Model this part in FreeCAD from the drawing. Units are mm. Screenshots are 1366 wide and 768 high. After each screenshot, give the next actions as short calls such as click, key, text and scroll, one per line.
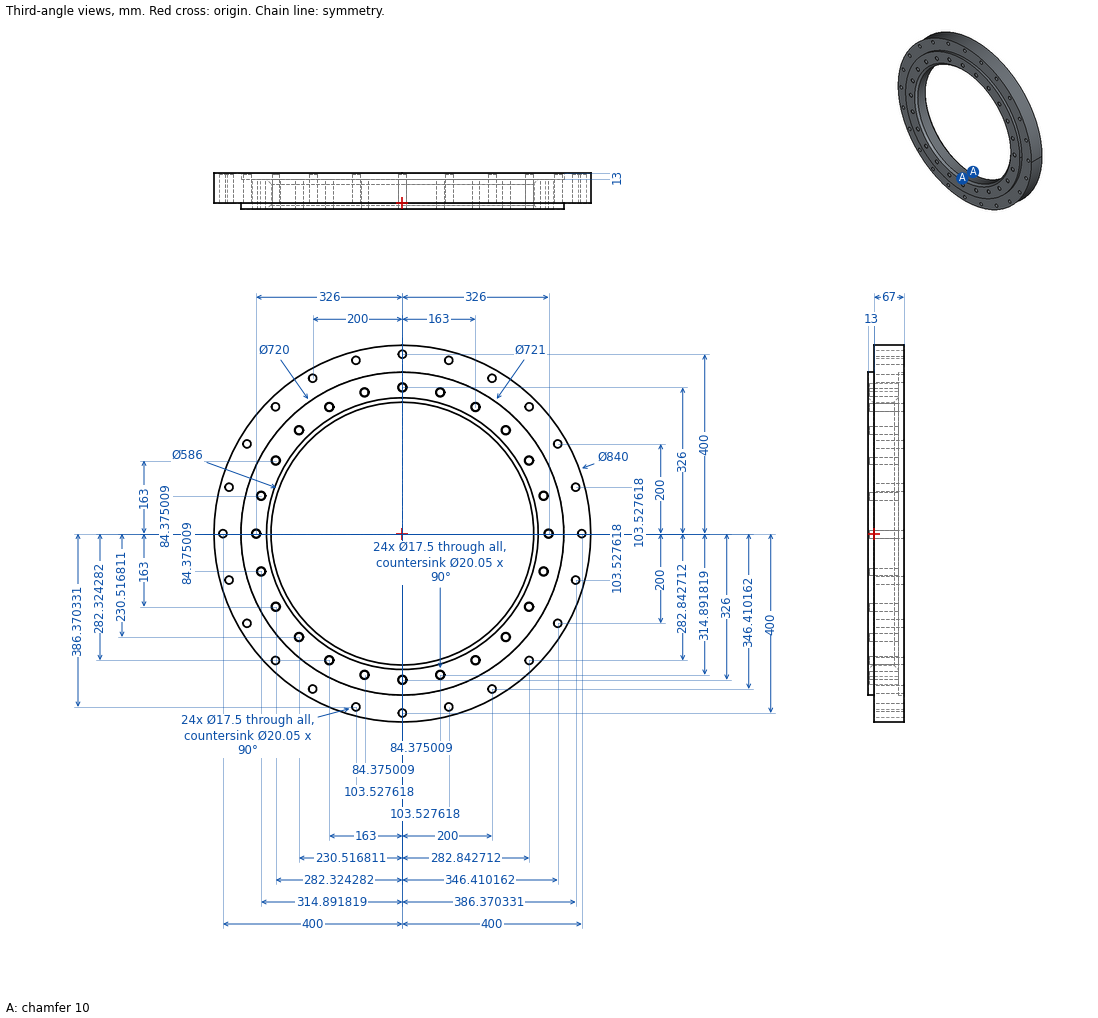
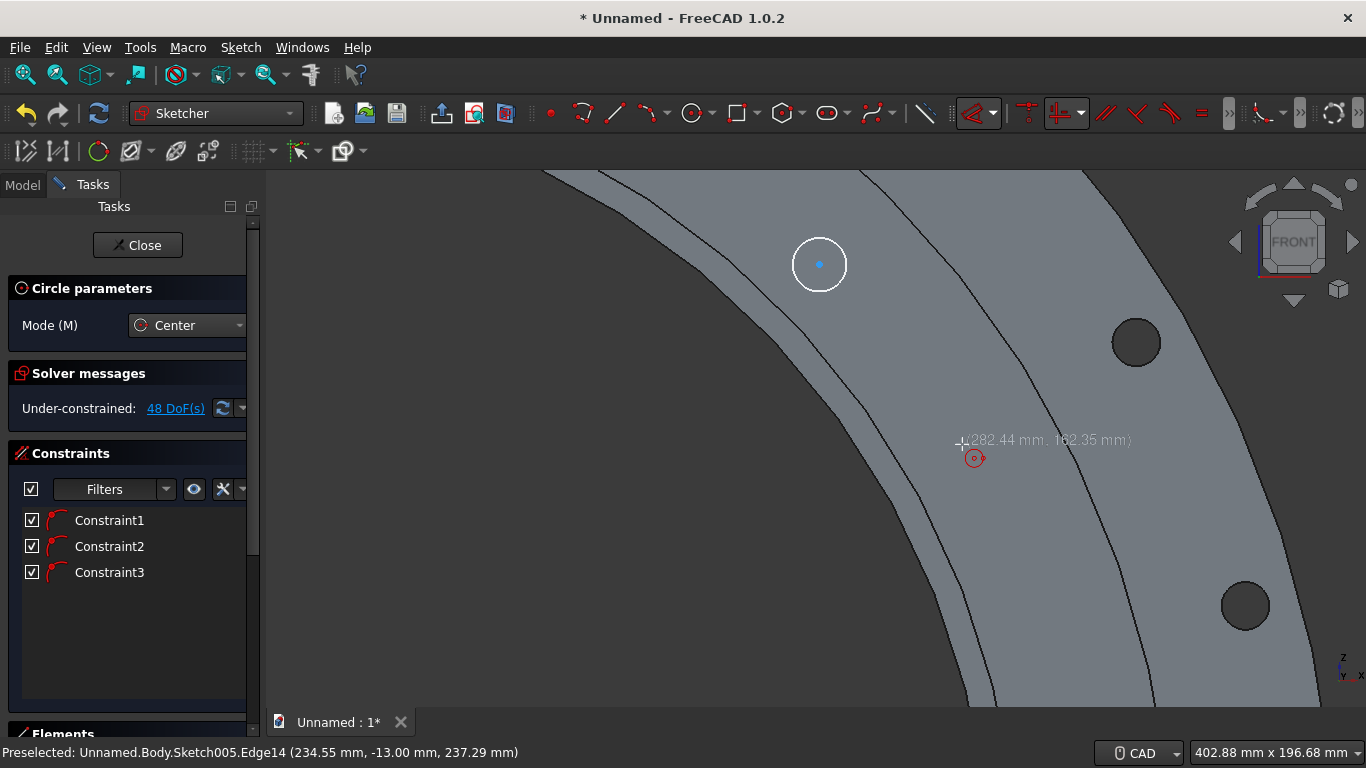
scroll(888, 325, down, 8)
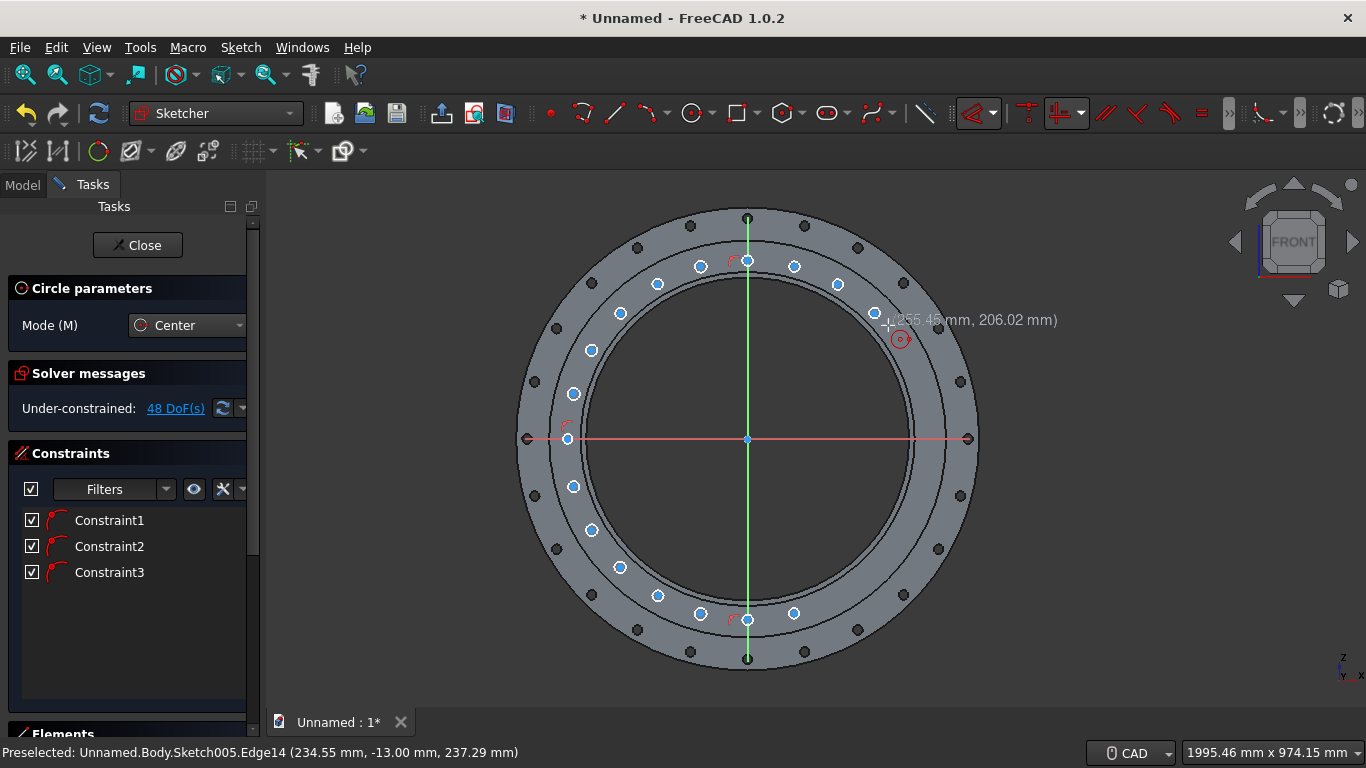
click(903, 349)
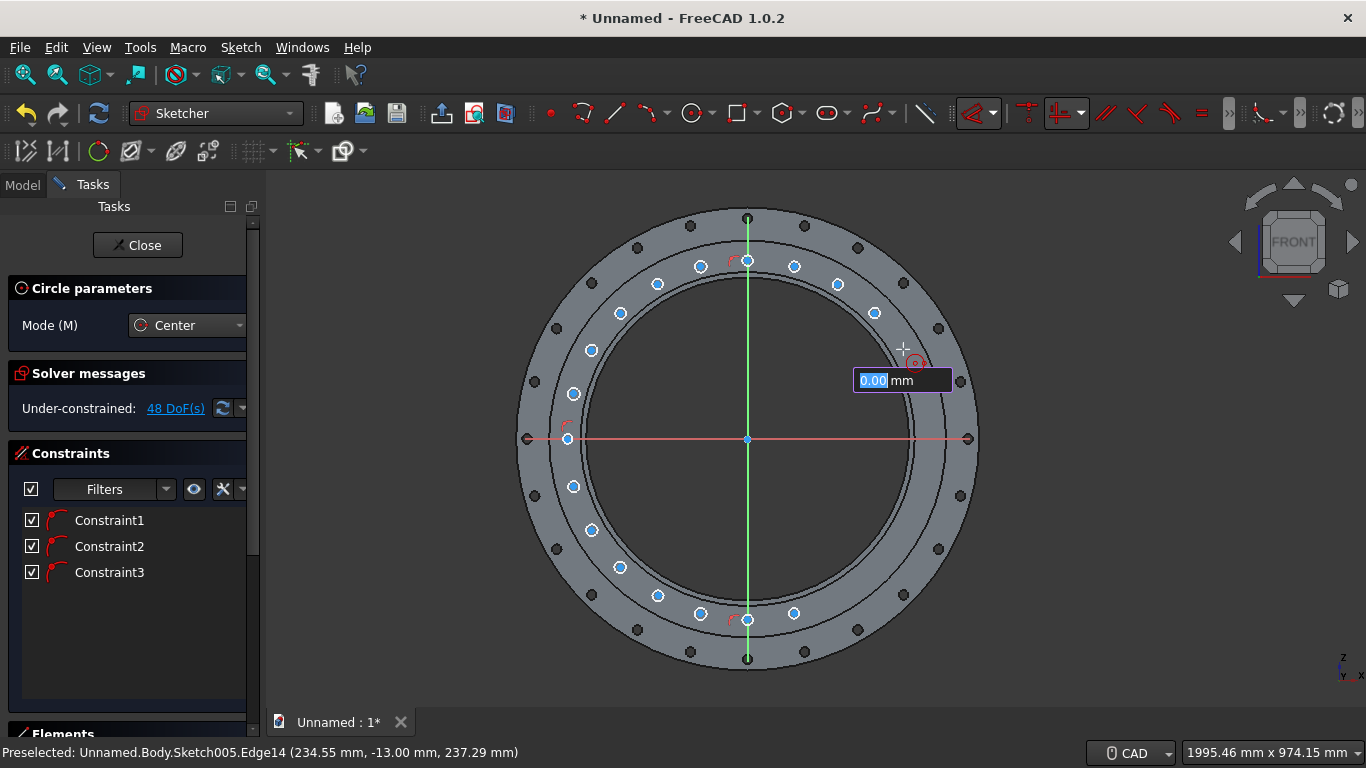
scroll(907, 346, up, 6)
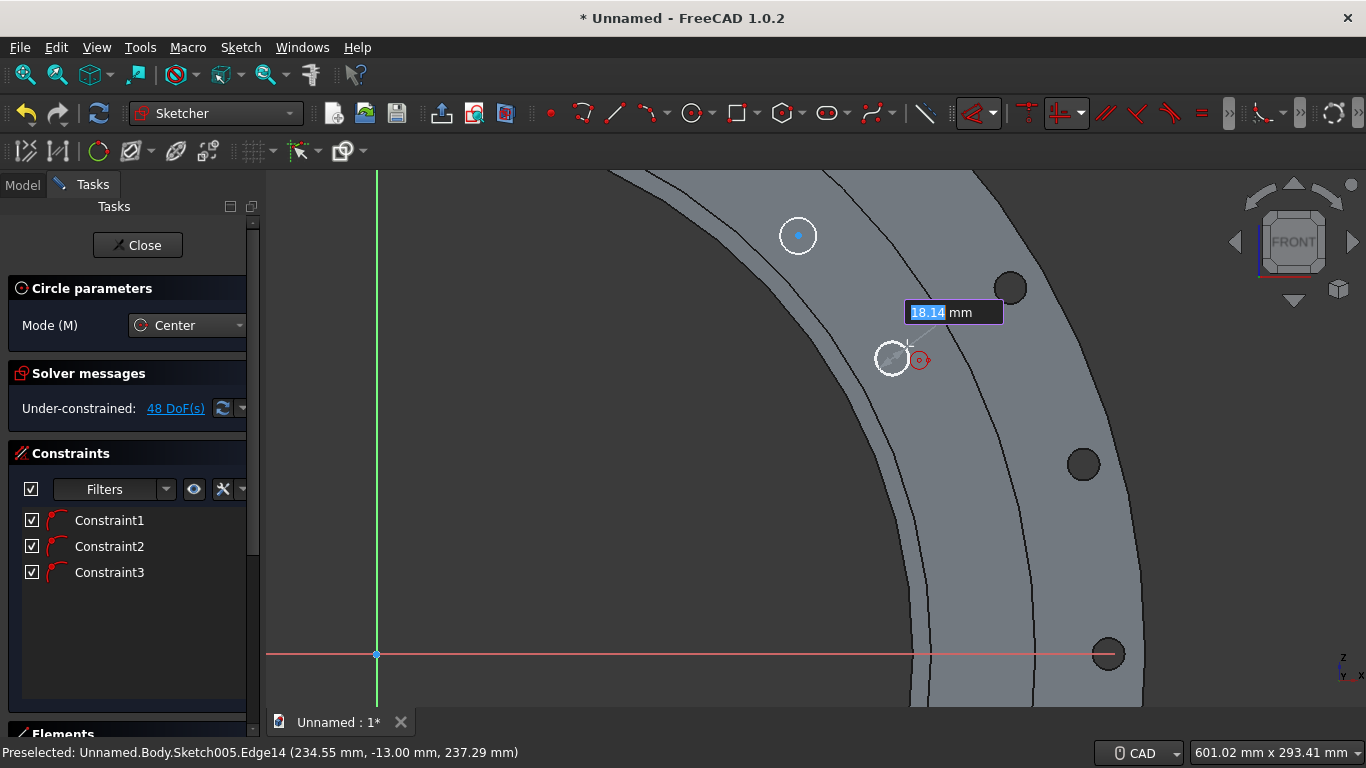
click(905, 344)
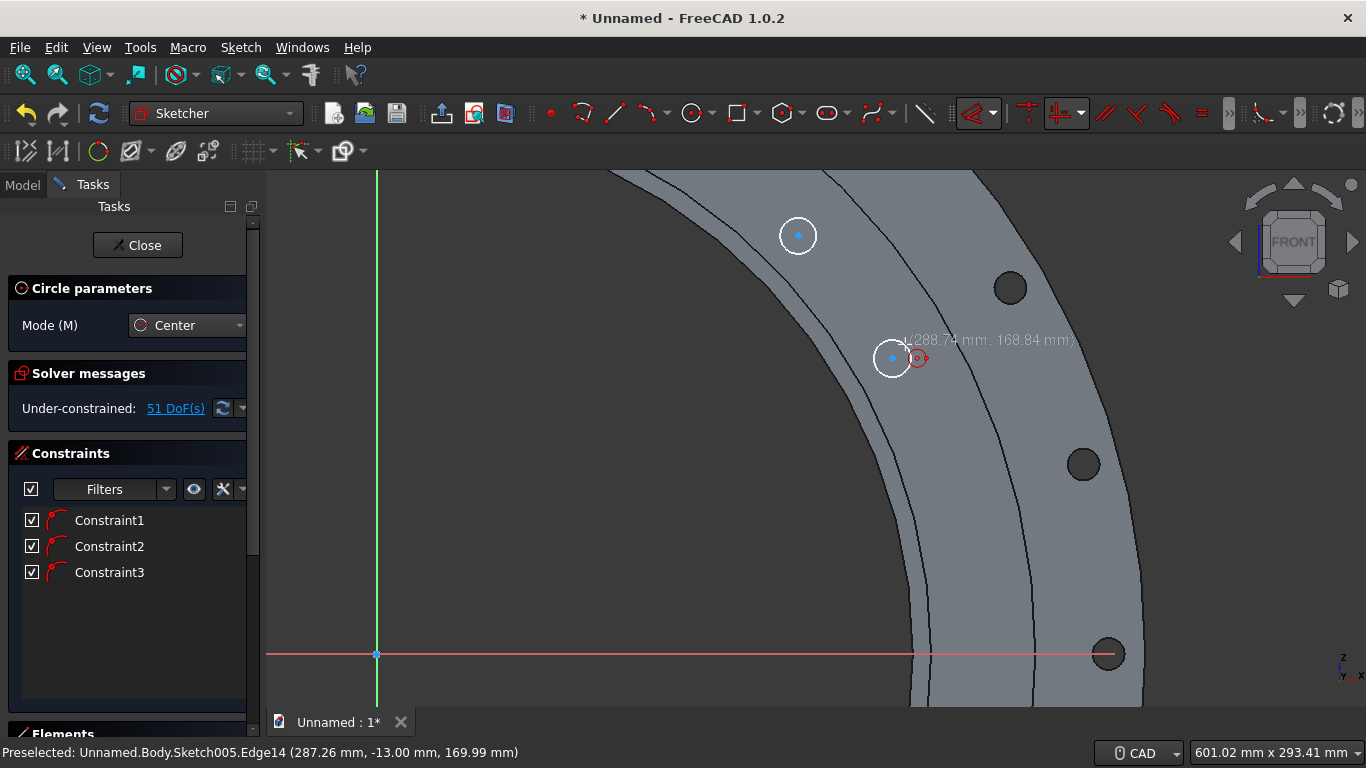
scroll(953, 500, up, 2)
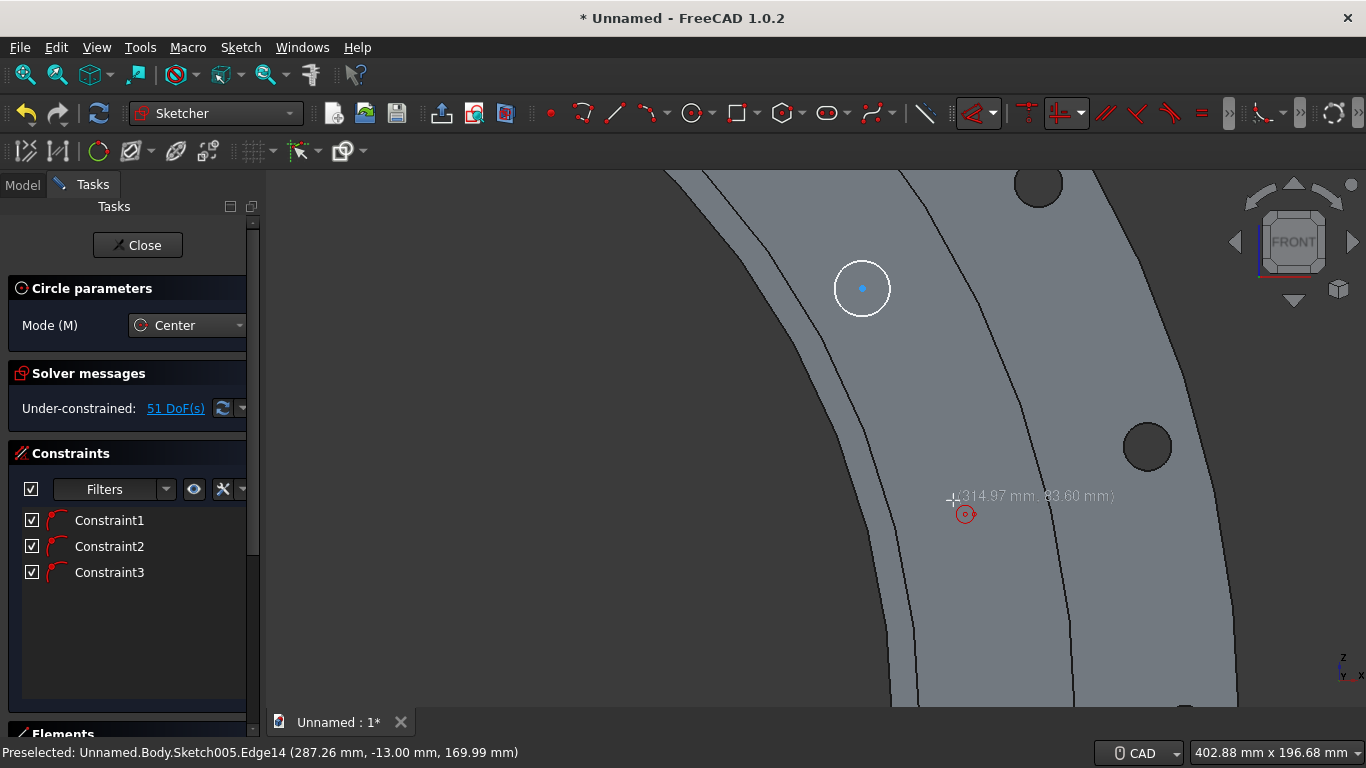
scroll(913, 365, down, 8)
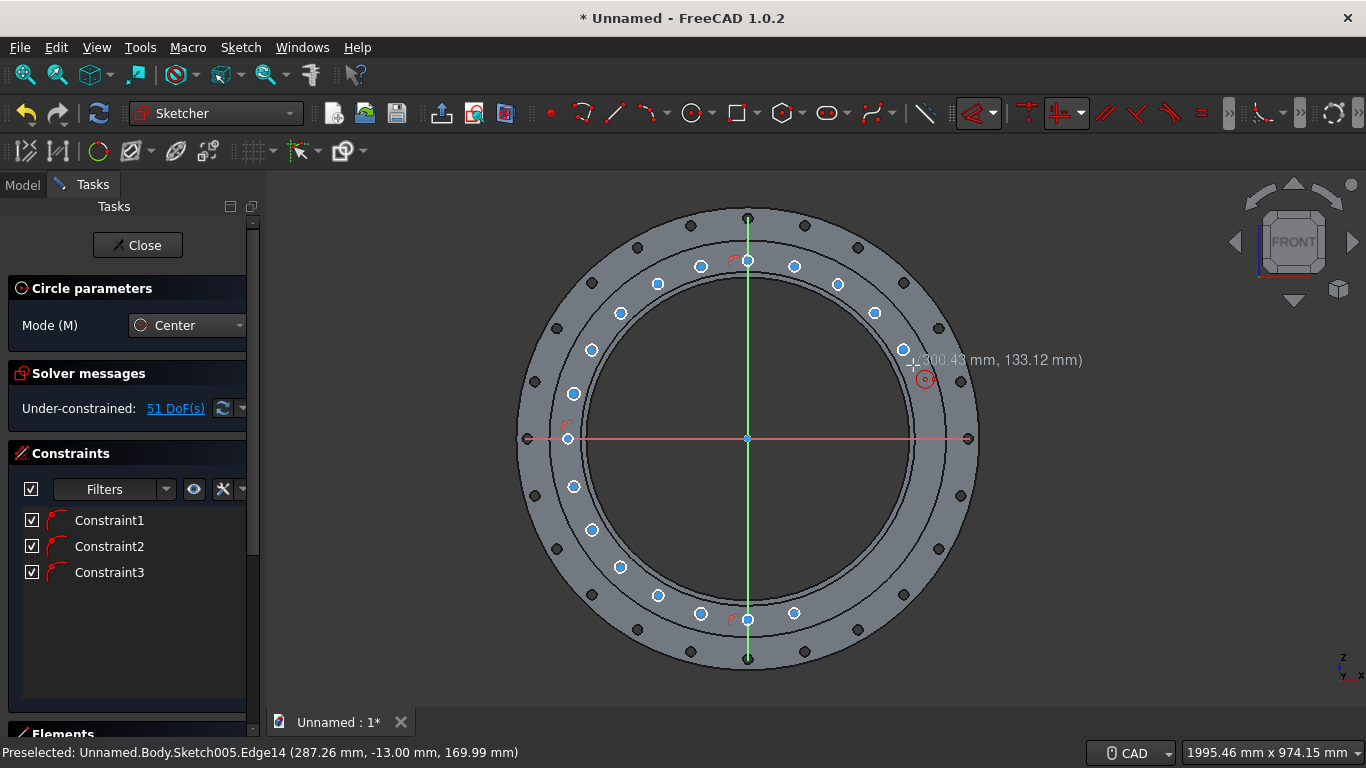
click(921, 392)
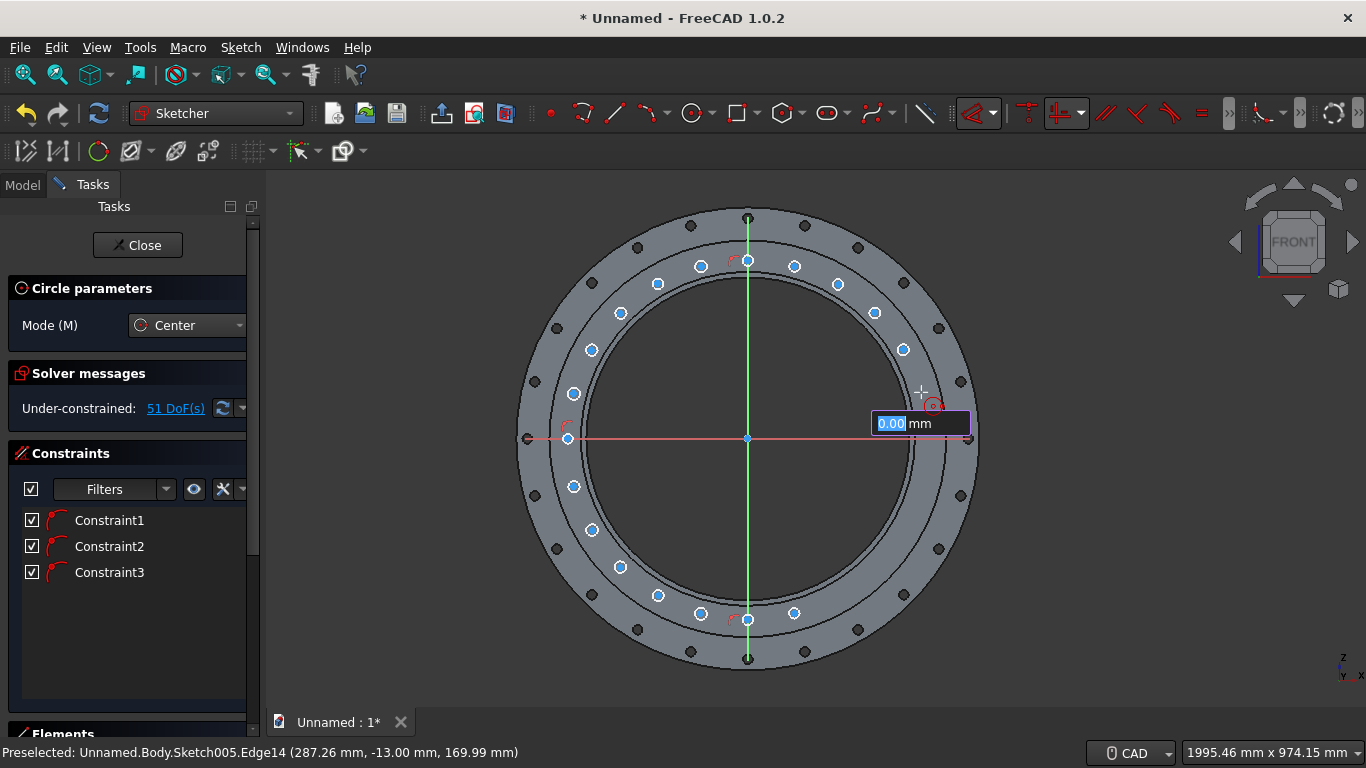
scroll(925, 389, up, 6)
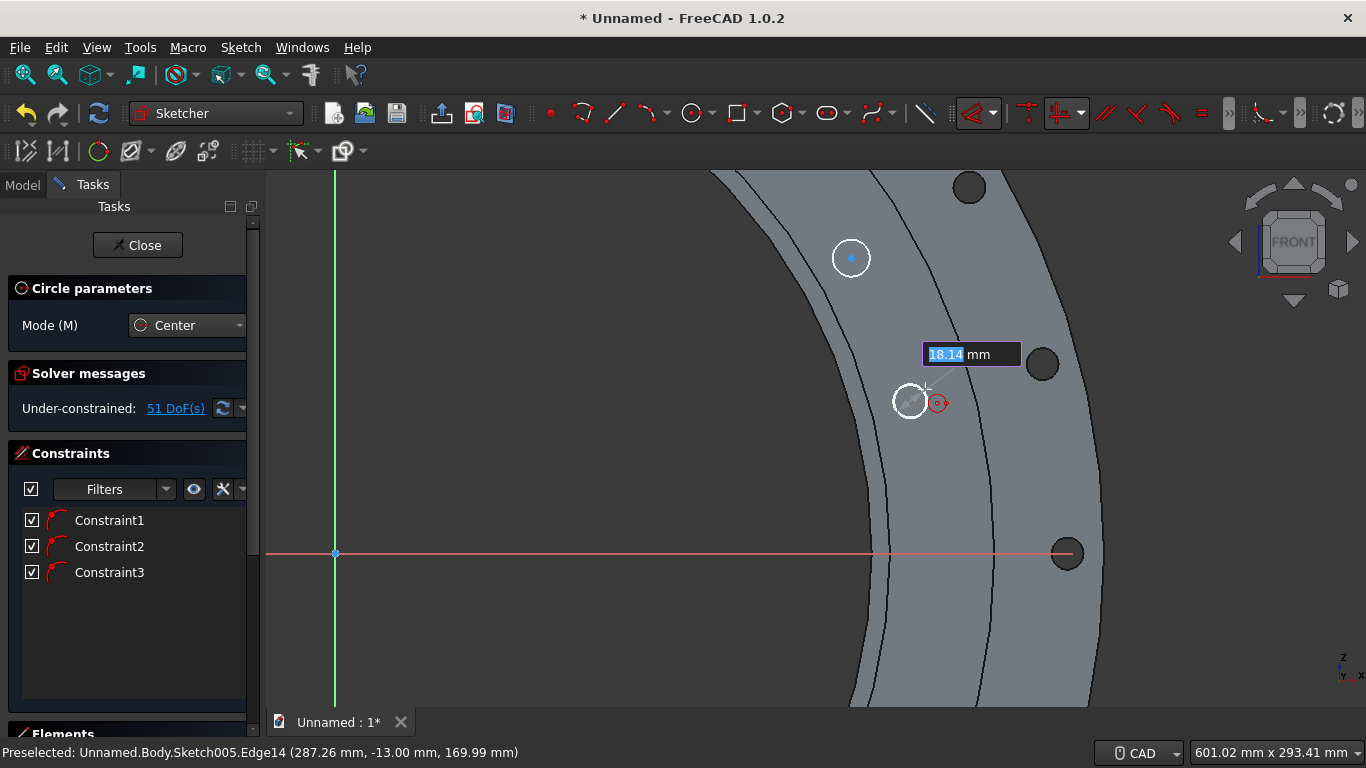
click(923, 388)